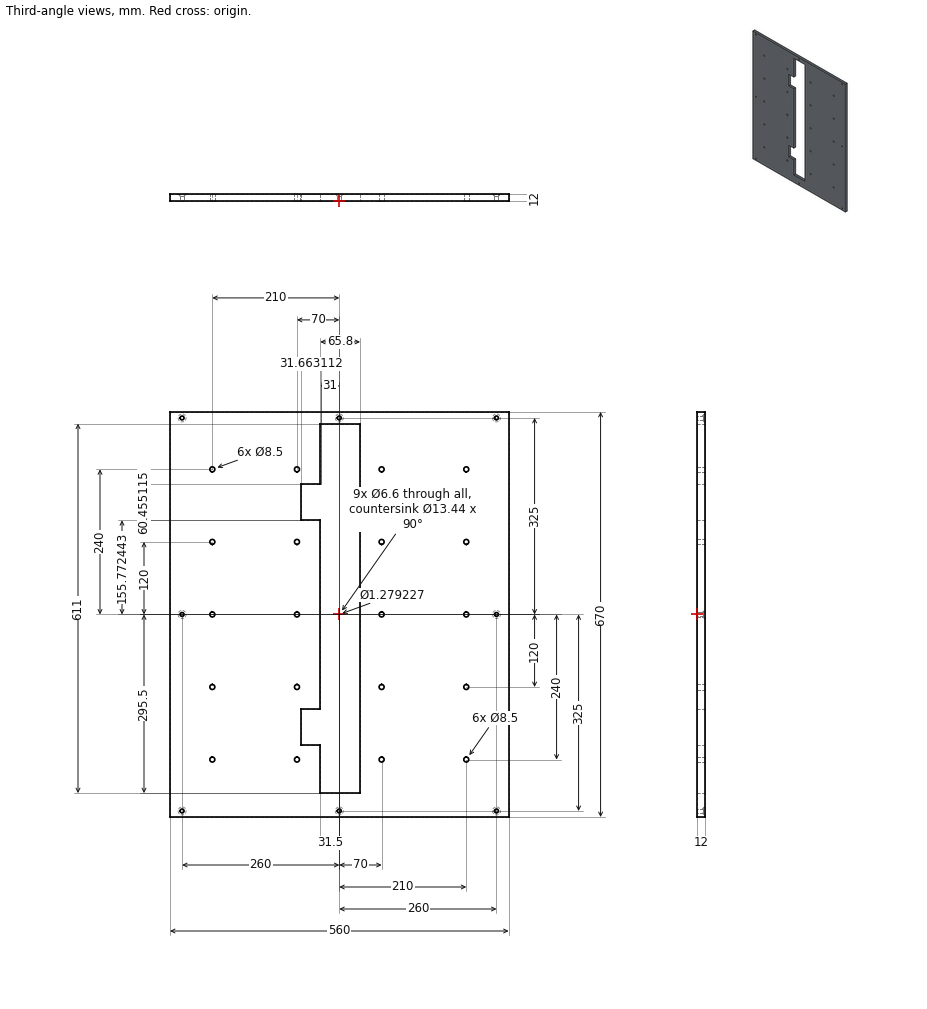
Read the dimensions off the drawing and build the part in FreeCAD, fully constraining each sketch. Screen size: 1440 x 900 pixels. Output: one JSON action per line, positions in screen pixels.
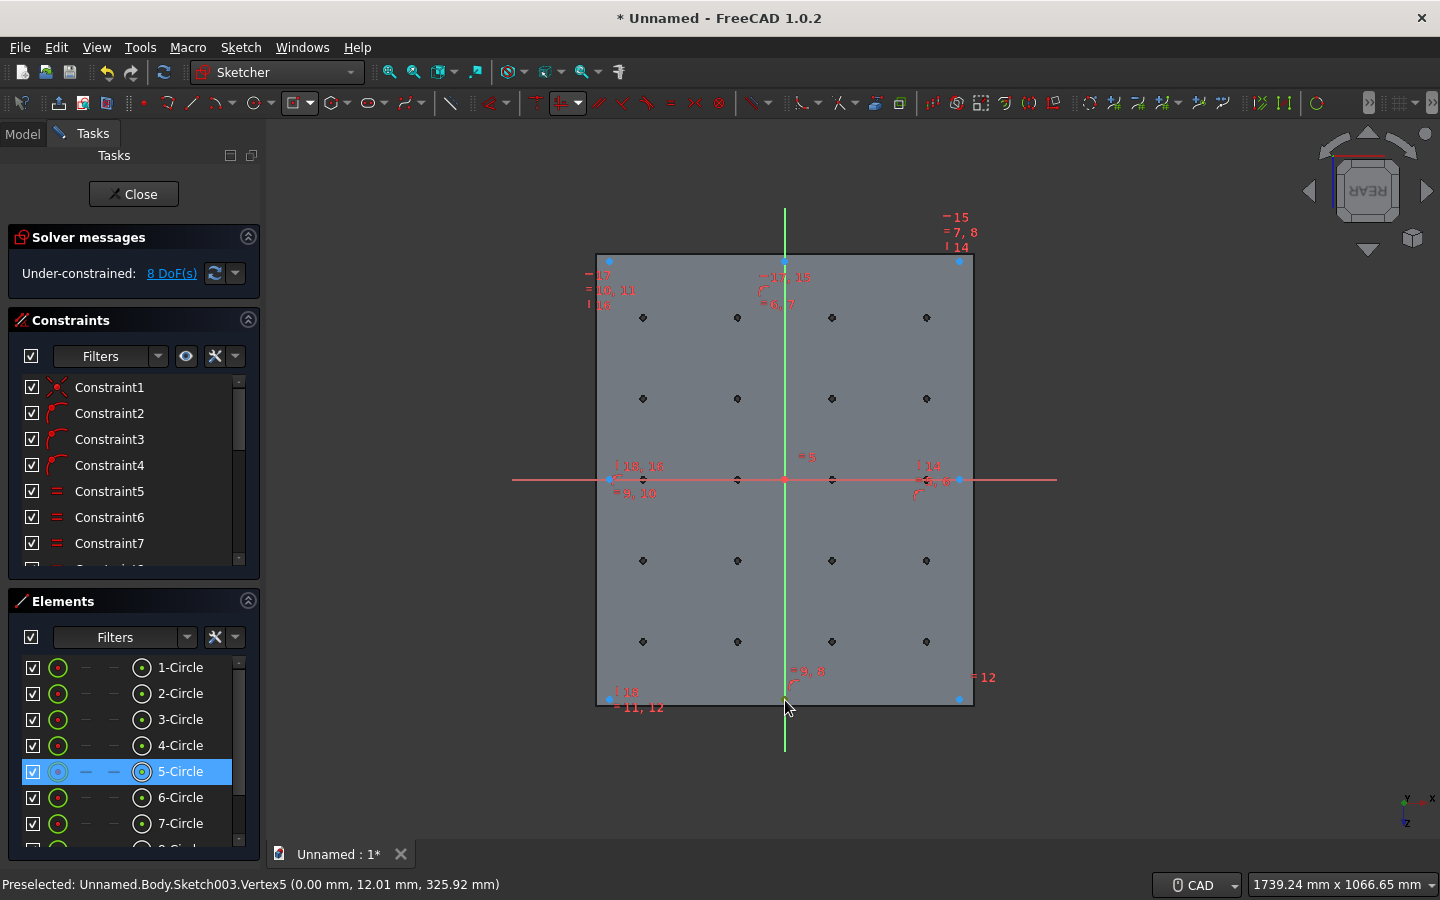
{"action": "left_click", "coordinate": [609, 700]}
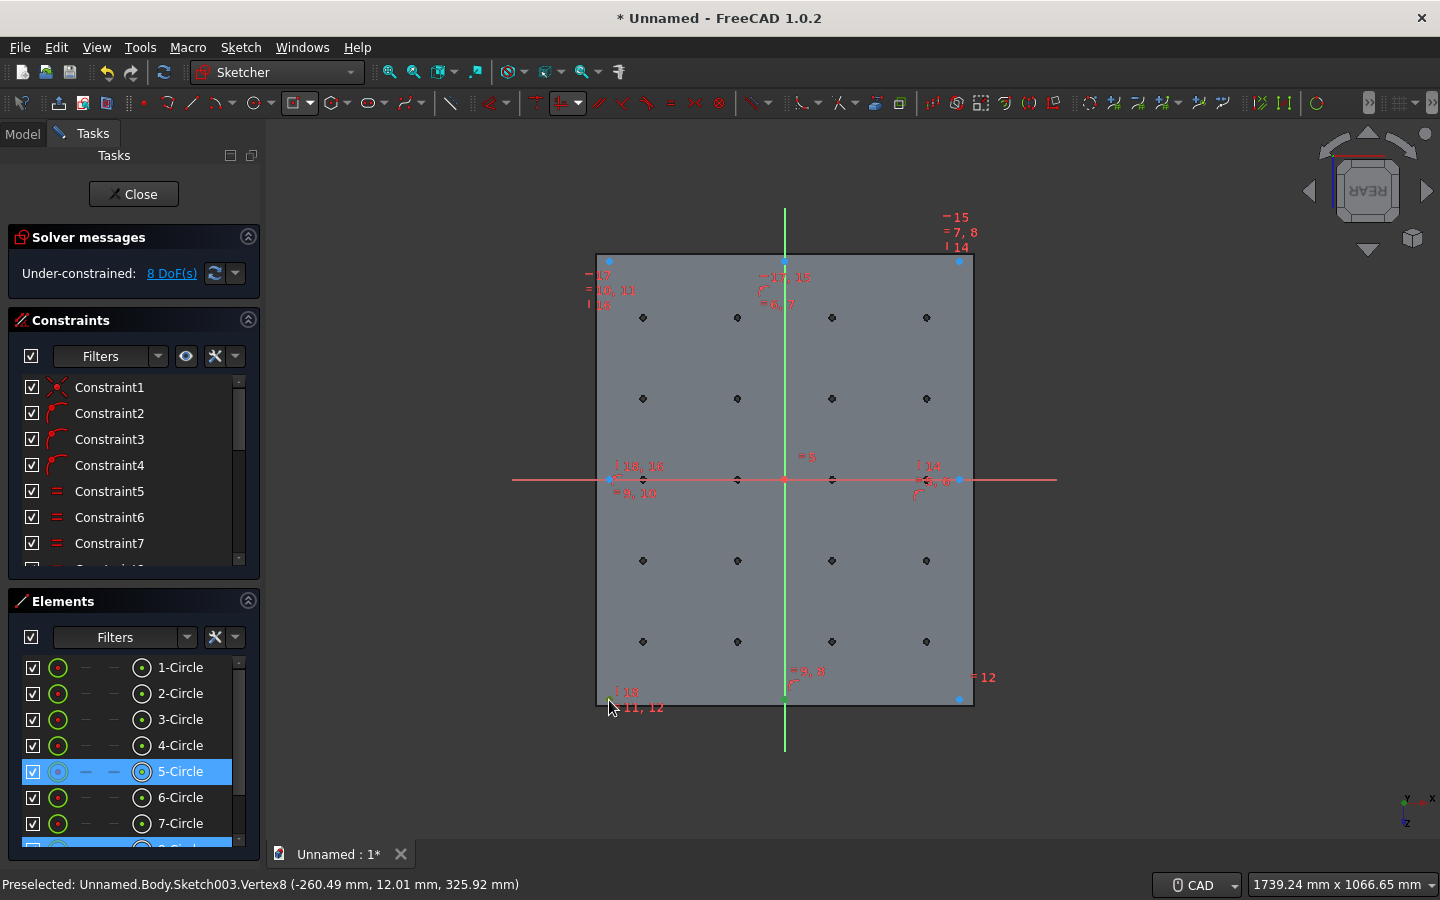
{"action": "key", "text": "h"}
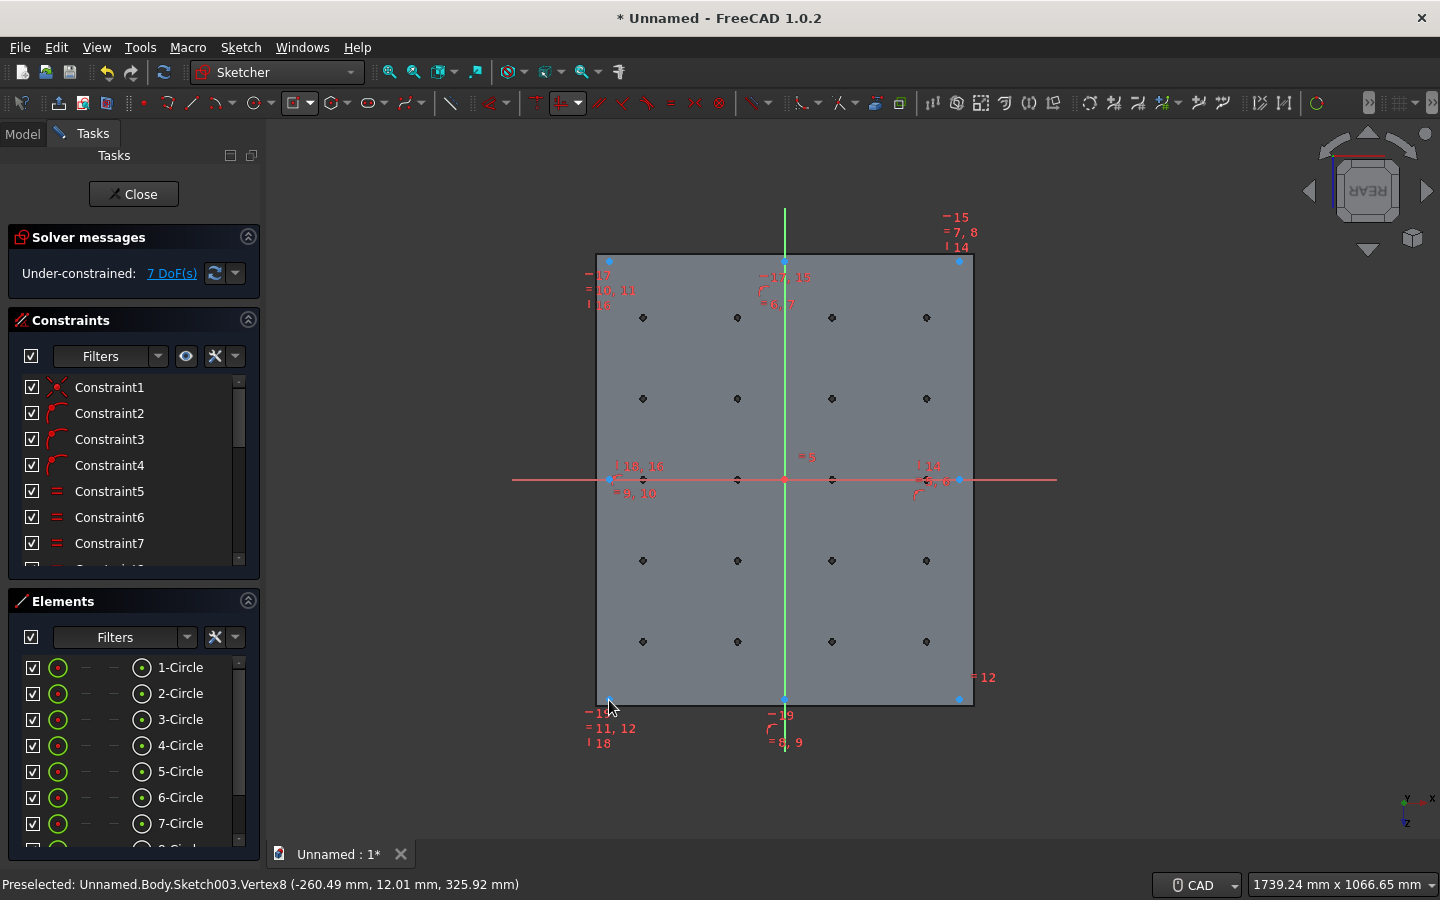
{"action": "left_click", "coordinate": [960, 480]}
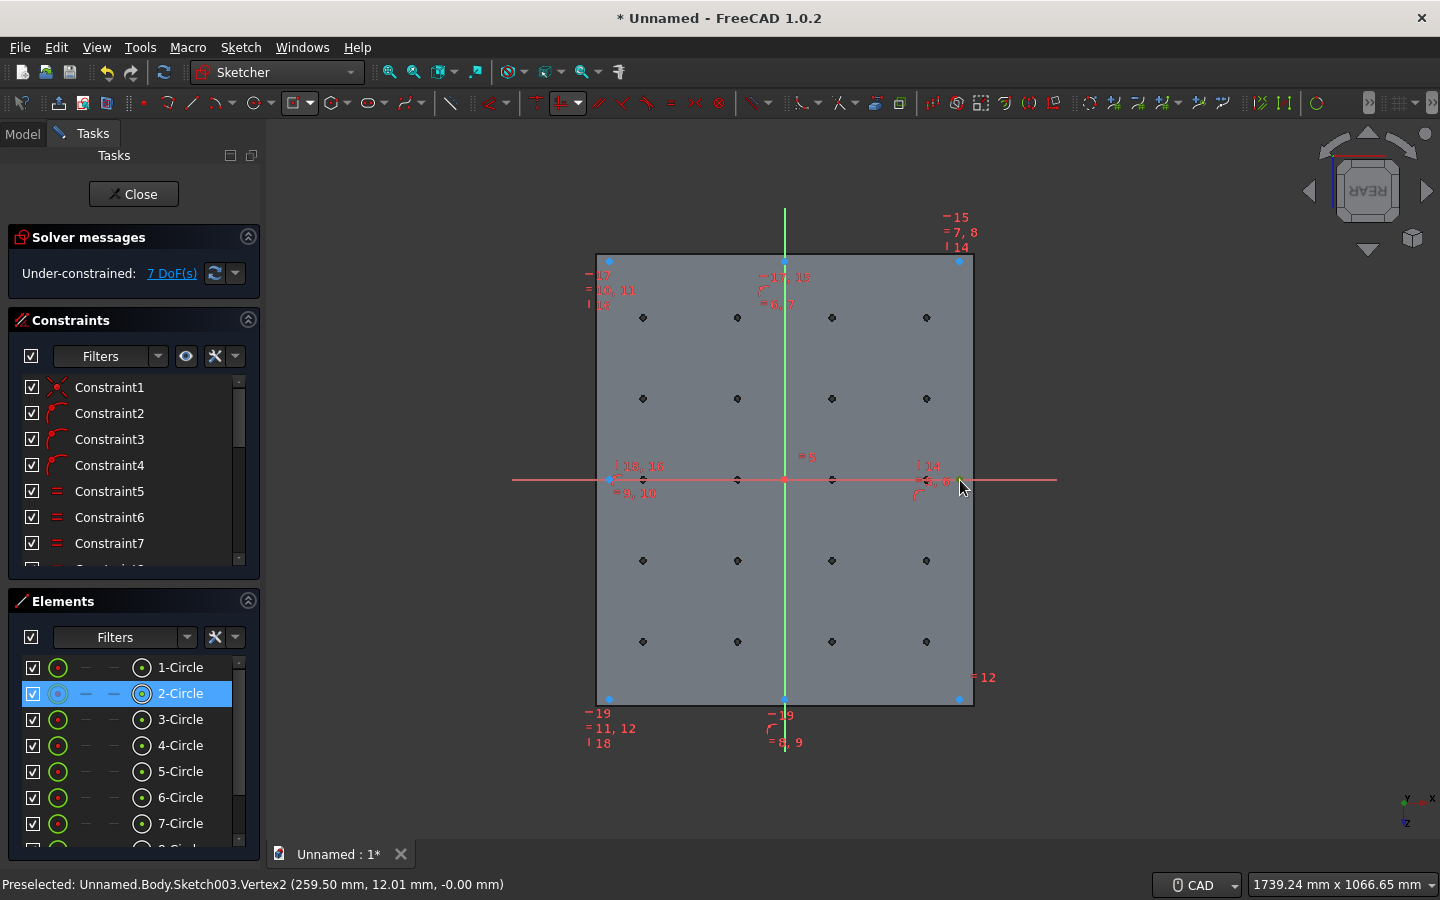
{"action": "left_click", "coordinate": [960, 700]}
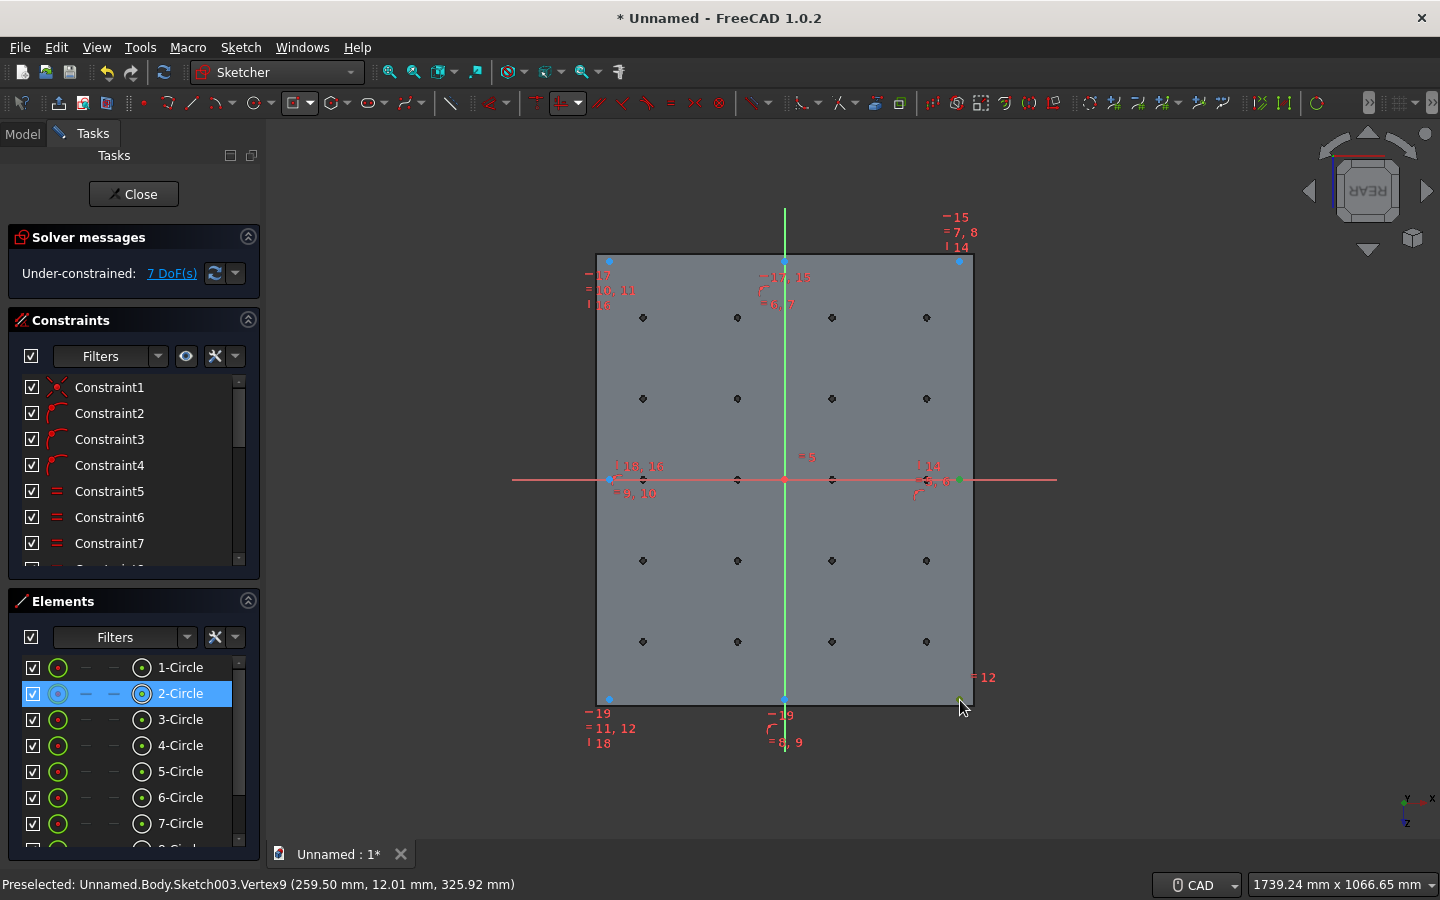
{"action": "left_click", "coordinate": [580, 104]}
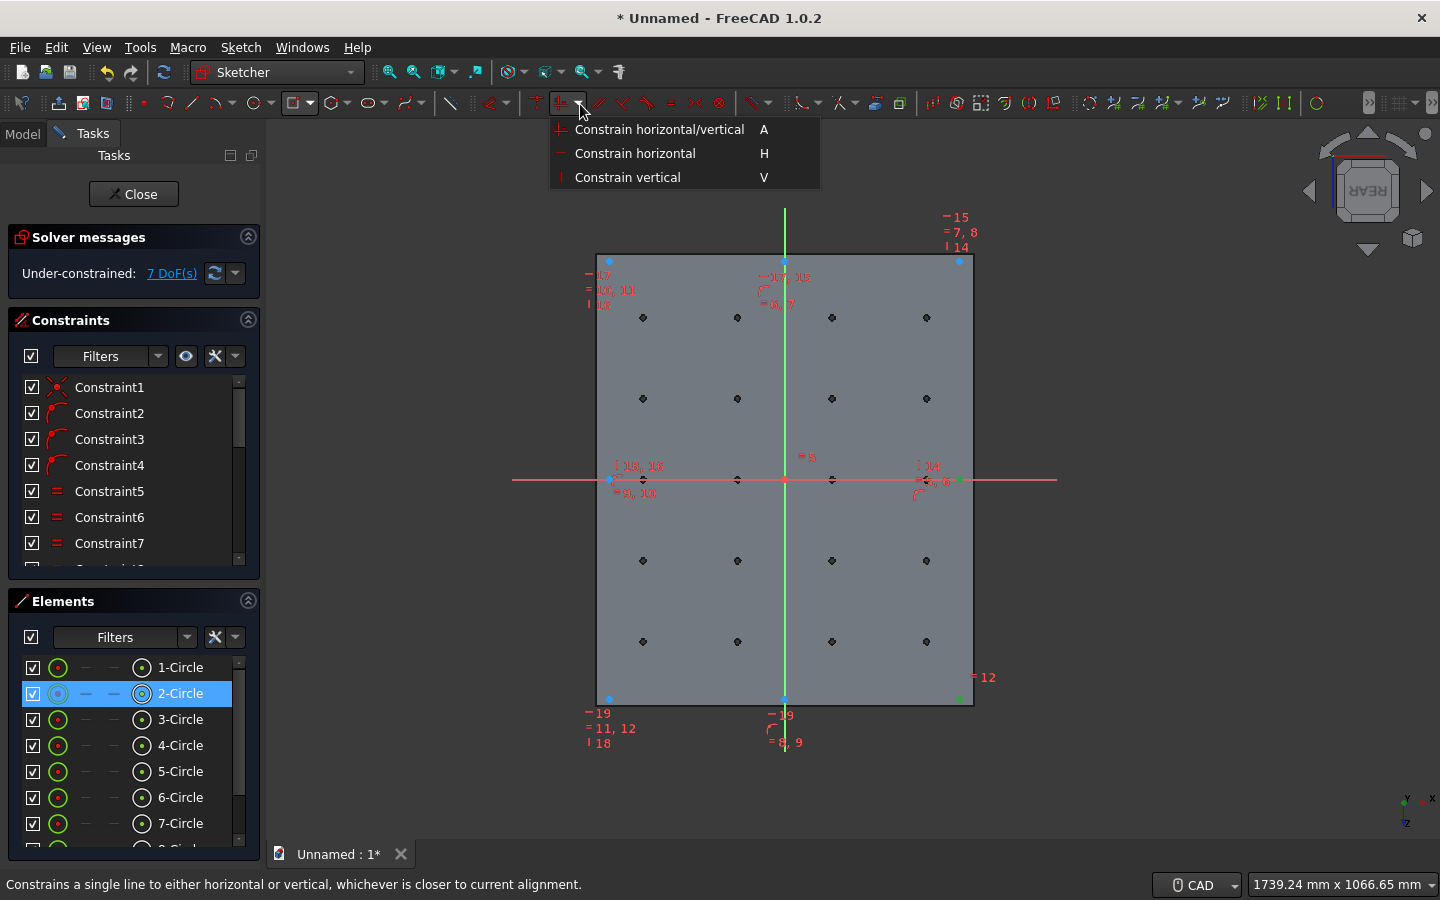
{"action": "left_click", "coordinate": [685, 177]}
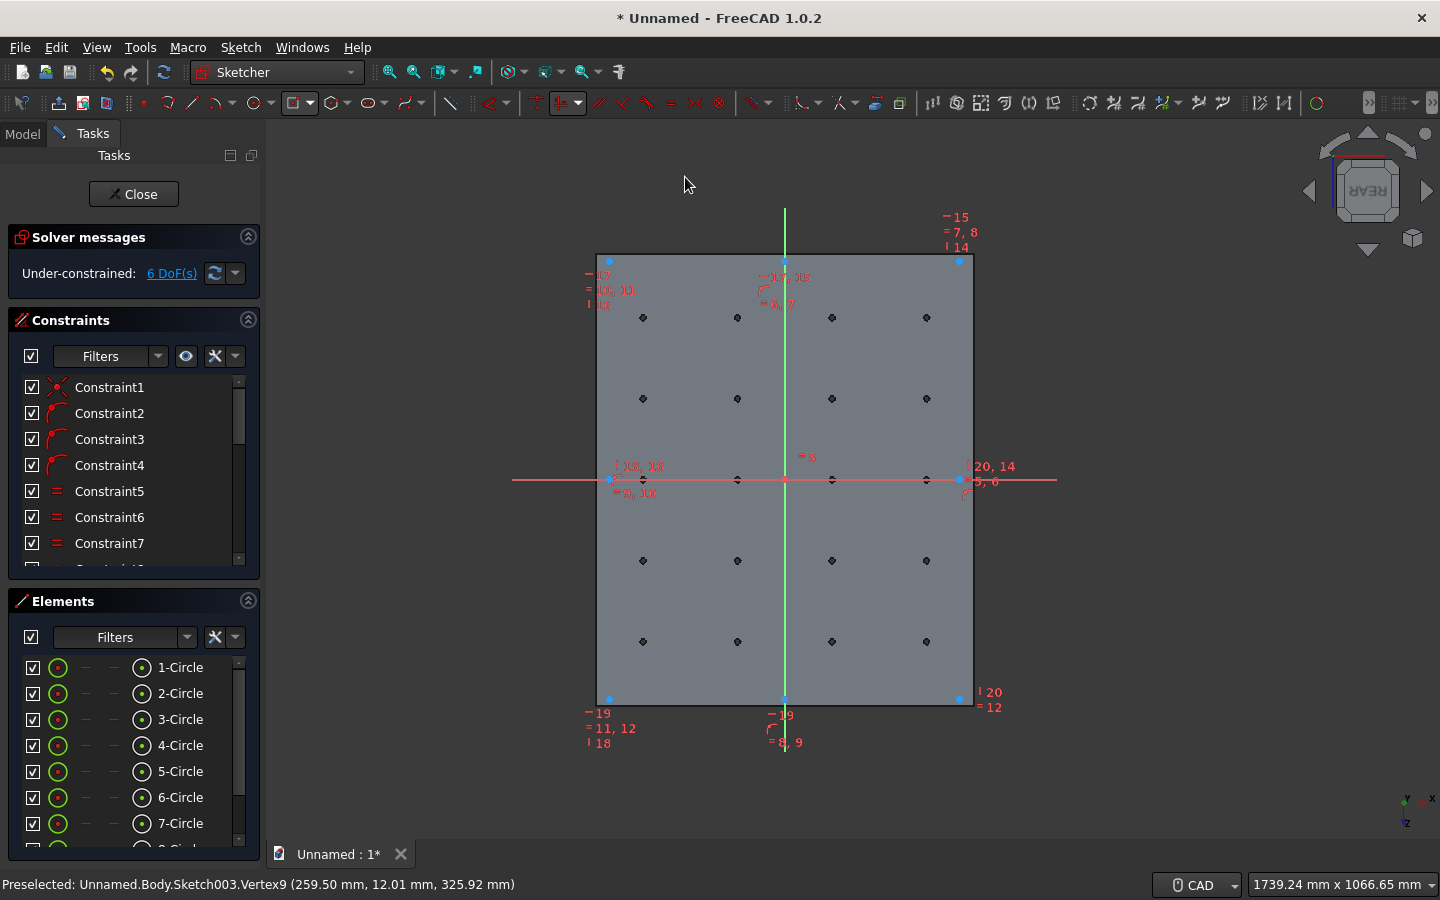
{"action": "left_click", "coordinate": [785, 700]}